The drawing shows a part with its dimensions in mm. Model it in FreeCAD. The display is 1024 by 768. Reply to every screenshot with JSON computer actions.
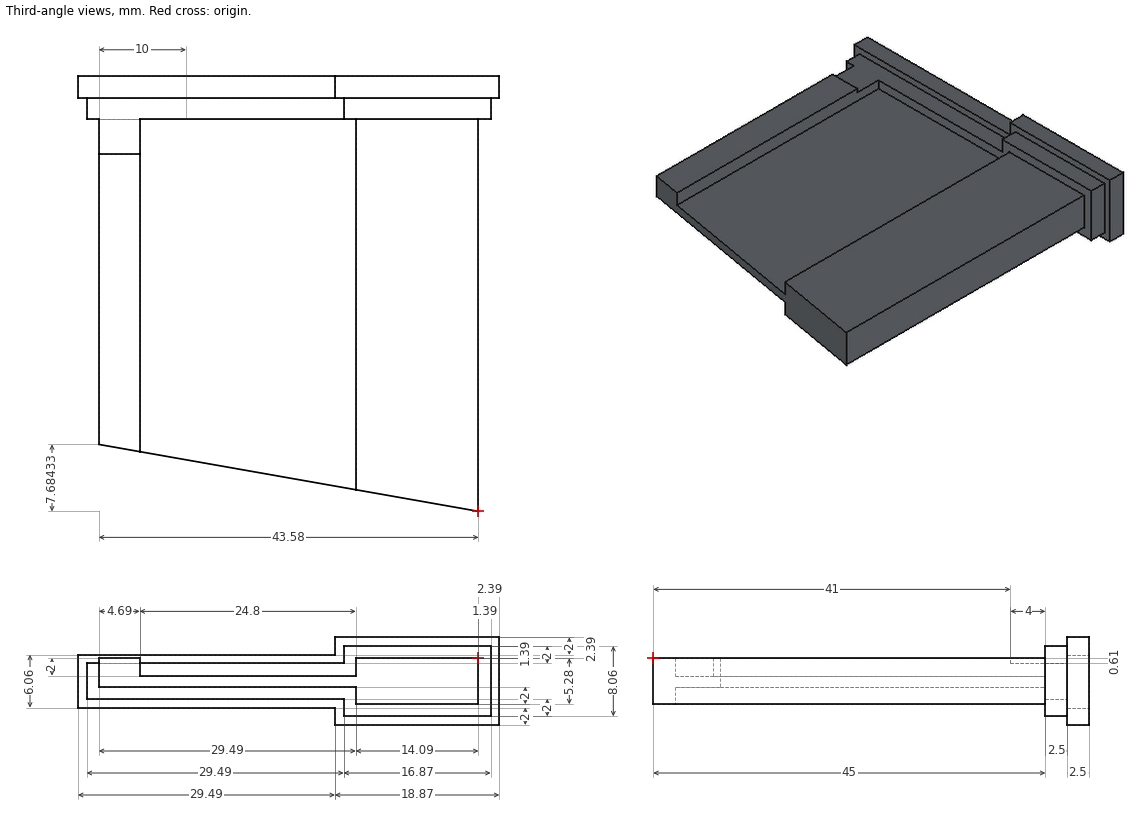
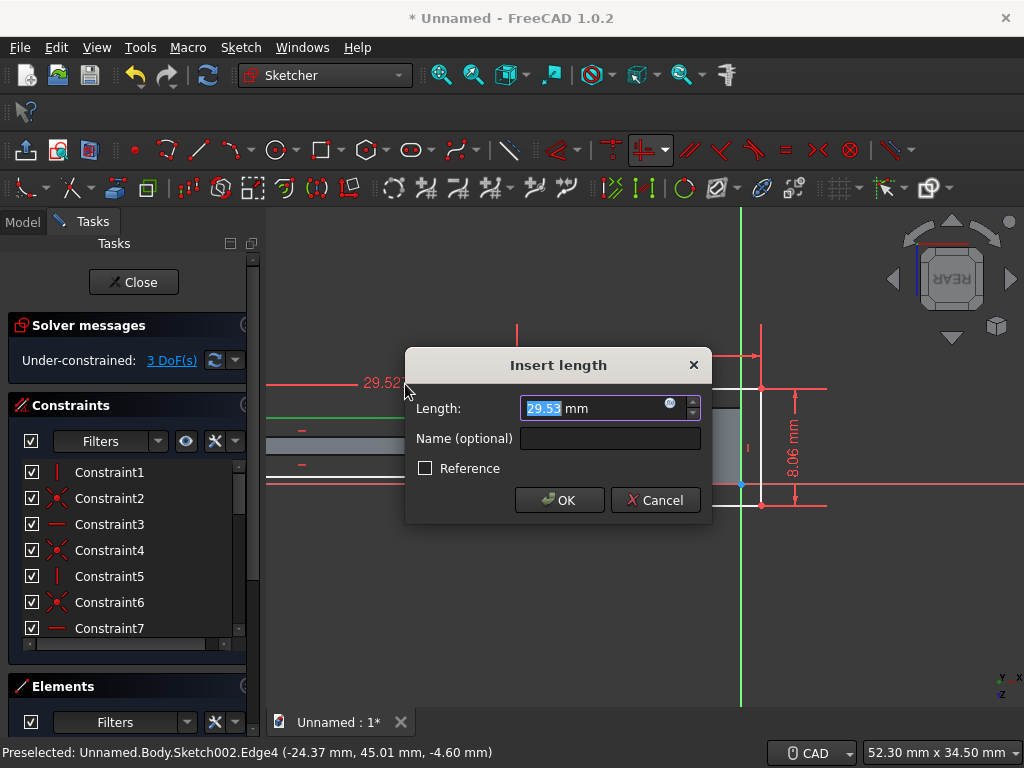
{"action": "type", "text": "29.49"}
{"action": "key", "text": "Return"}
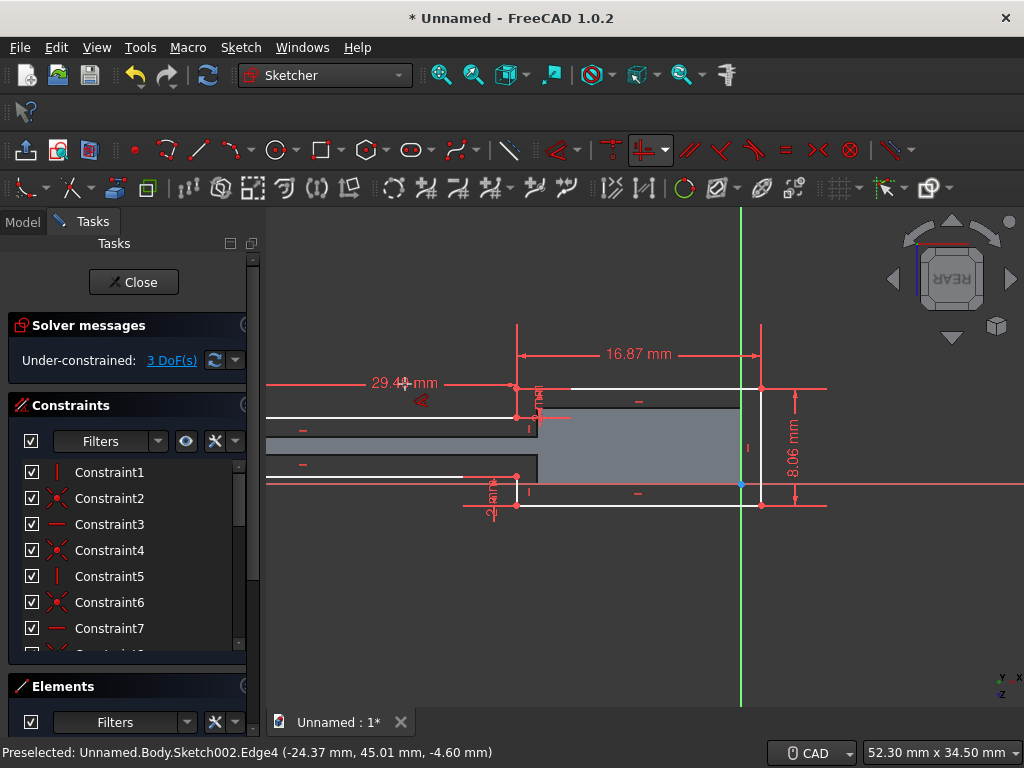
{"action": "scroll", "coordinate": [388, 477], "scroll_direction": "up", "scroll_amount": 3}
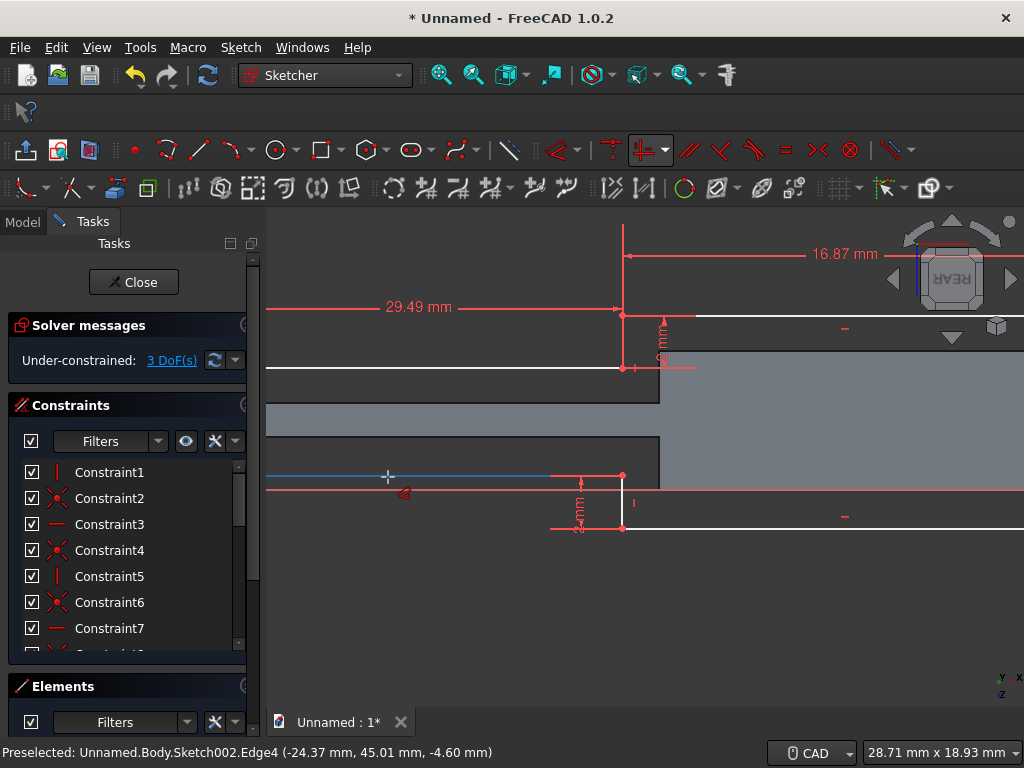
{"action": "left_click", "coordinate": [389, 476]}
{"action": "left_click", "coordinate": [458, 510]}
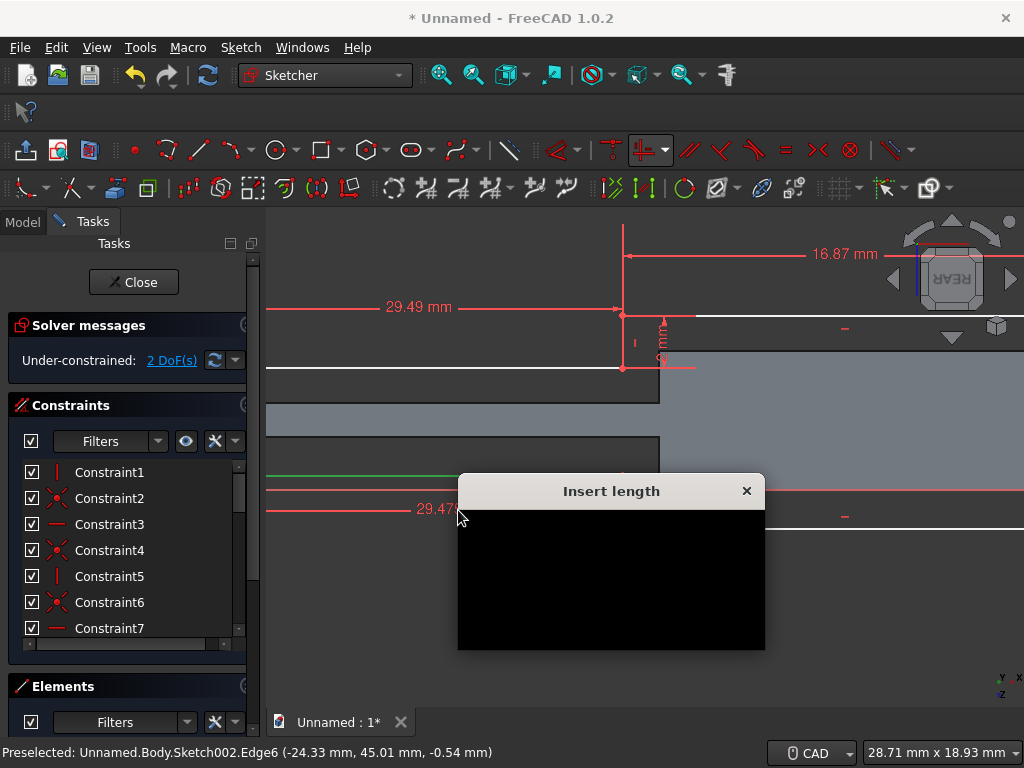
{"action": "type", "text": "29.49"}
{"action": "key", "text": "Return"}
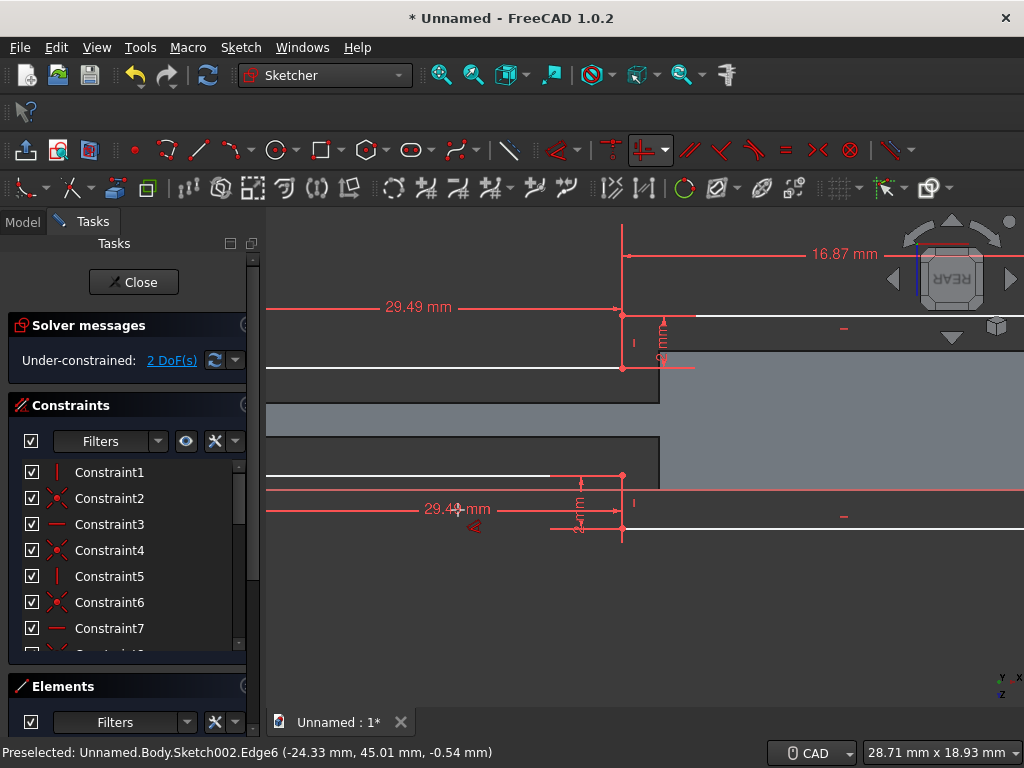
{"action": "scroll", "coordinate": [628, 473], "scroll_direction": "down", "scroll_amount": 6}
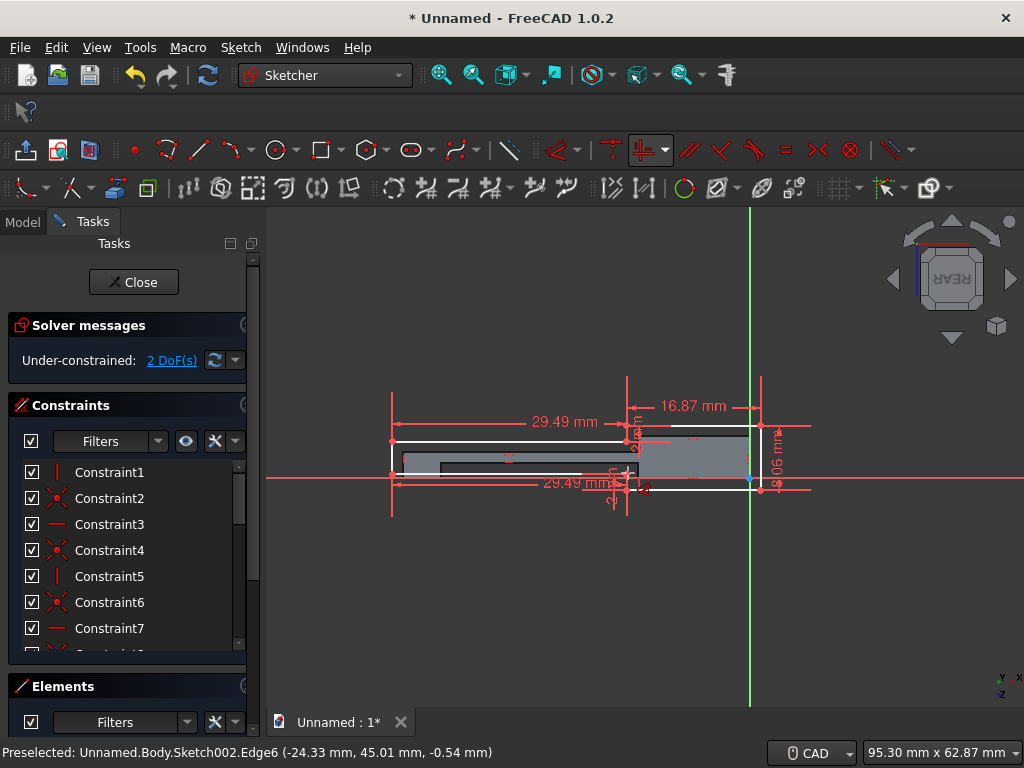
{"action": "scroll", "coordinate": [761, 490], "scroll_direction": "up", "scroll_amount": 7}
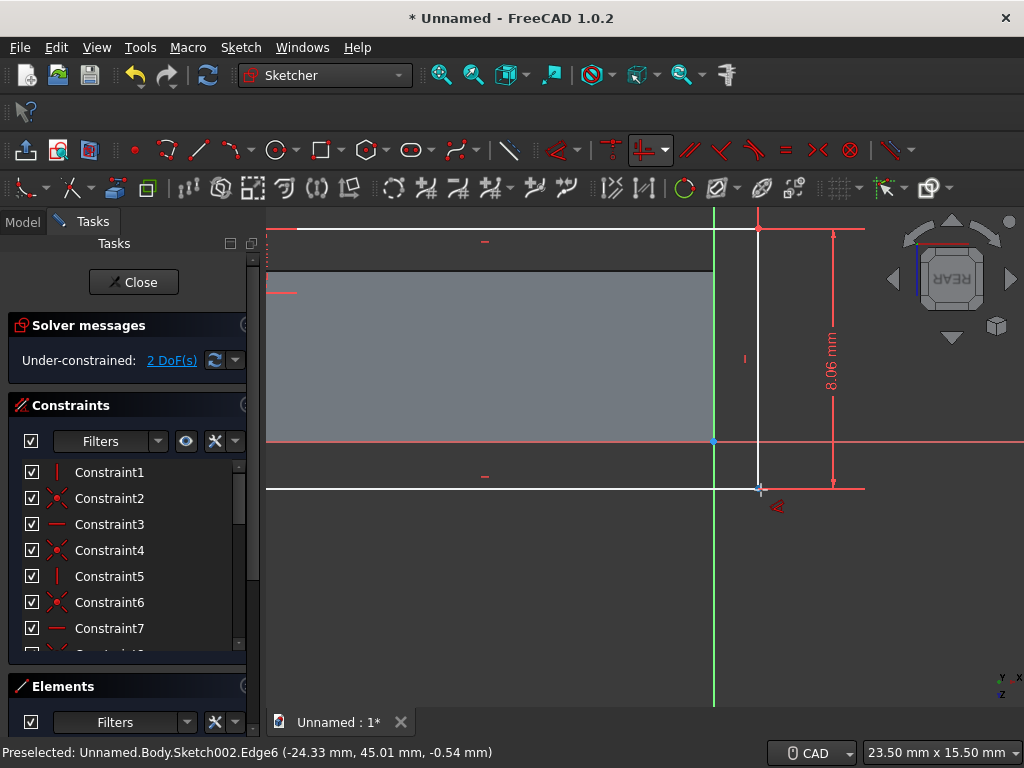
{"action": "left_click", "coordinate": [758, 489]}
{"action": "left_click", "coordinate": [736, 523]}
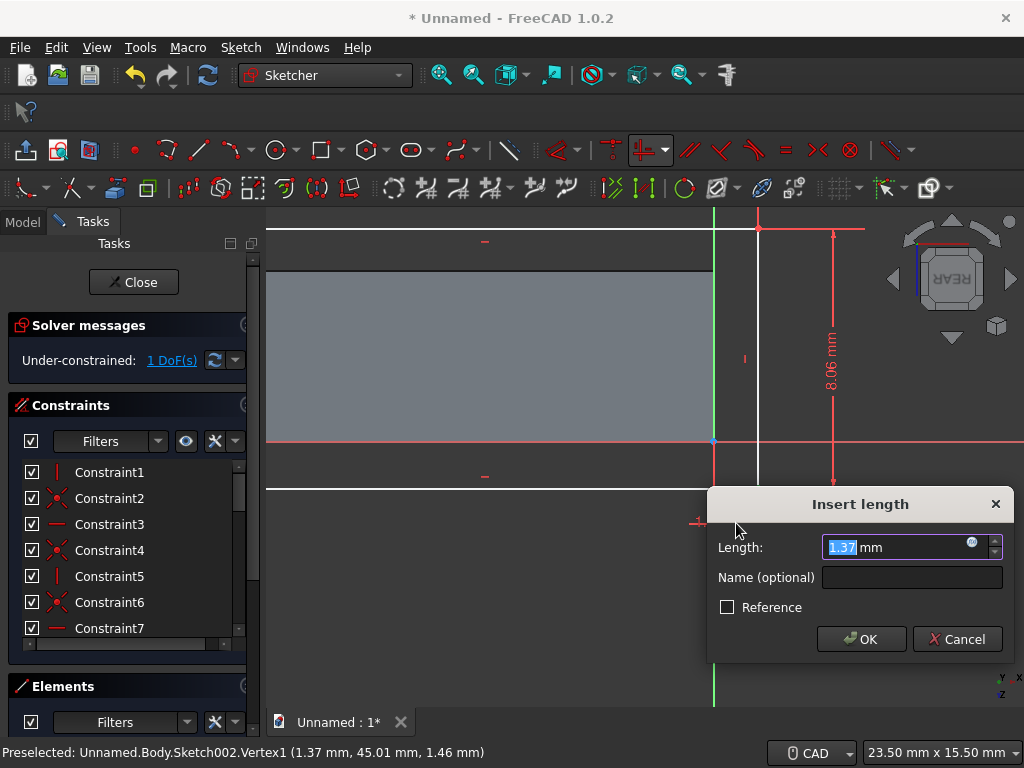
{"action": "type", "text": "1.39"}
{"action": "key", "text": "Return"}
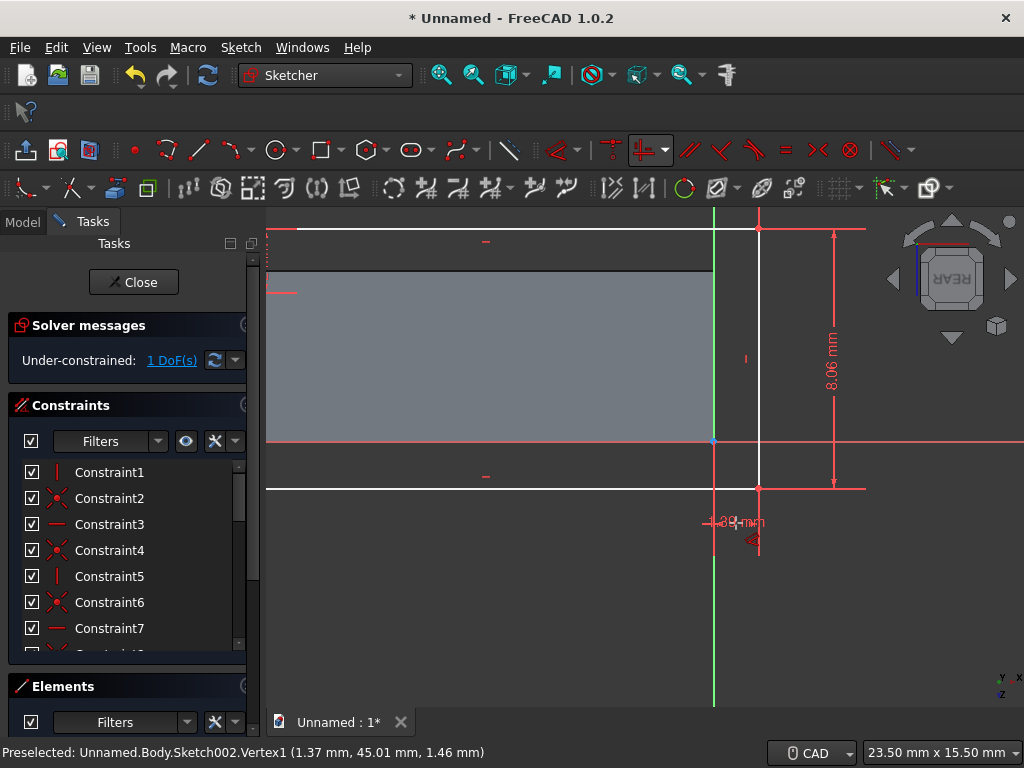
{"action": "left_click", "coordinate": [759, 489]}
{"action": "left_click", "coordinate": [793, 465]}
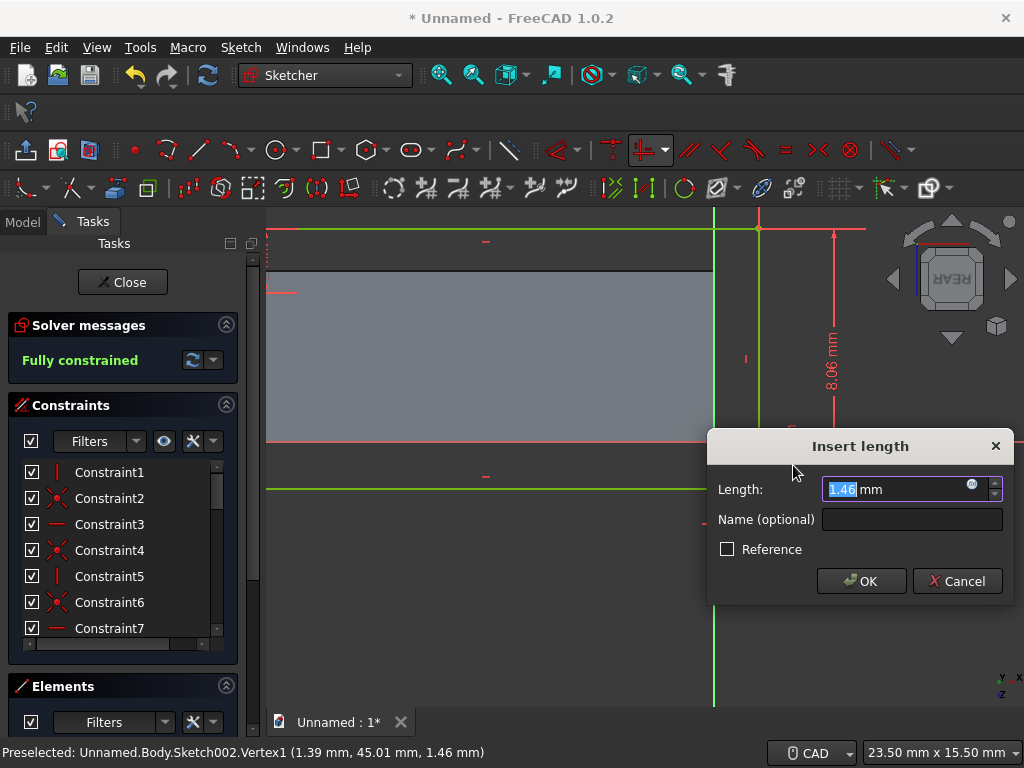
{"action": "type", "text": "1.39"}
{"action": "key", "text": "Return"}
{"action": "key", "text": "Escape"}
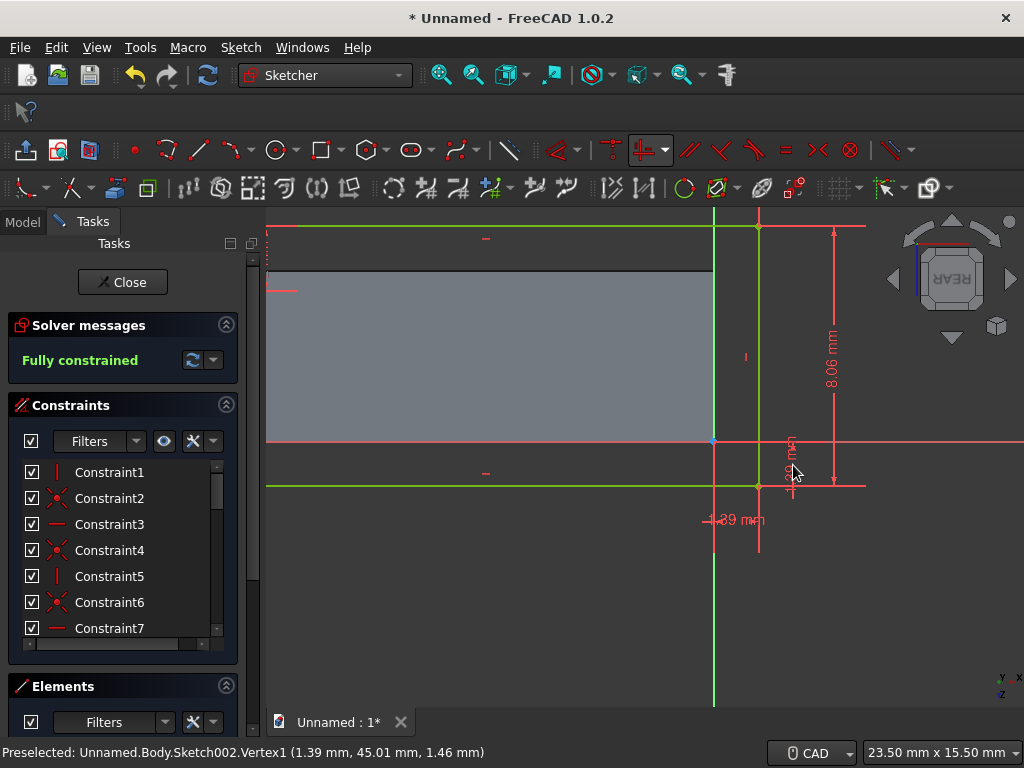
{"action": "left_click", "coordinate": [123, 282]}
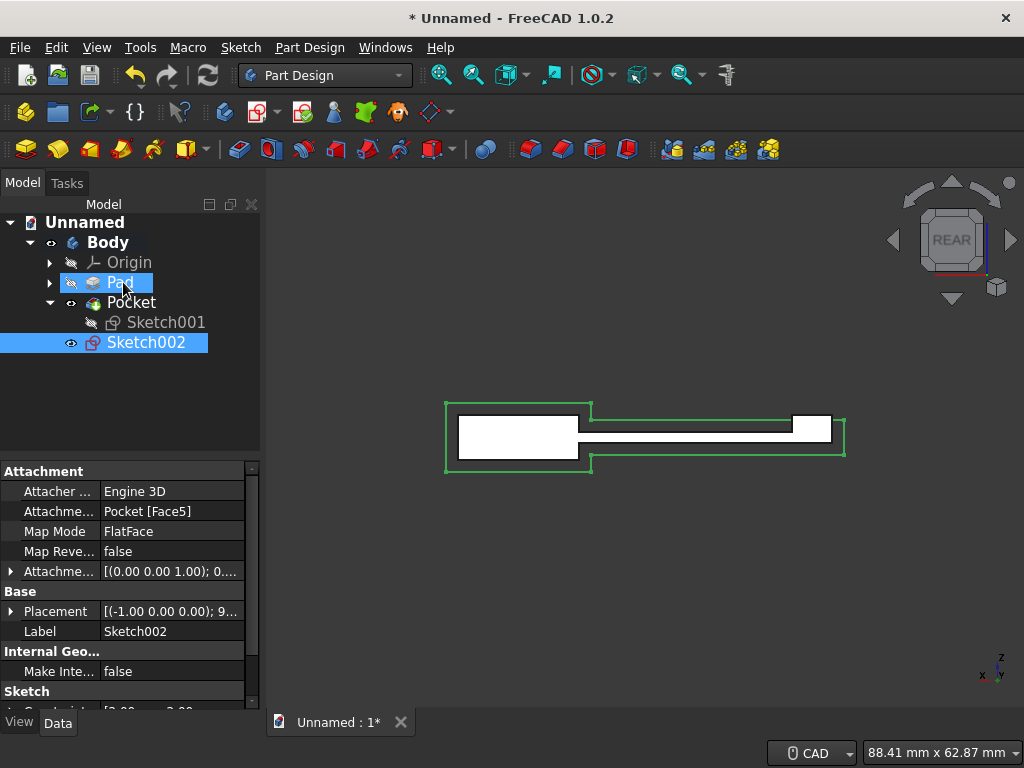
{"action": "left_click", "coordinate": [26, 150]}